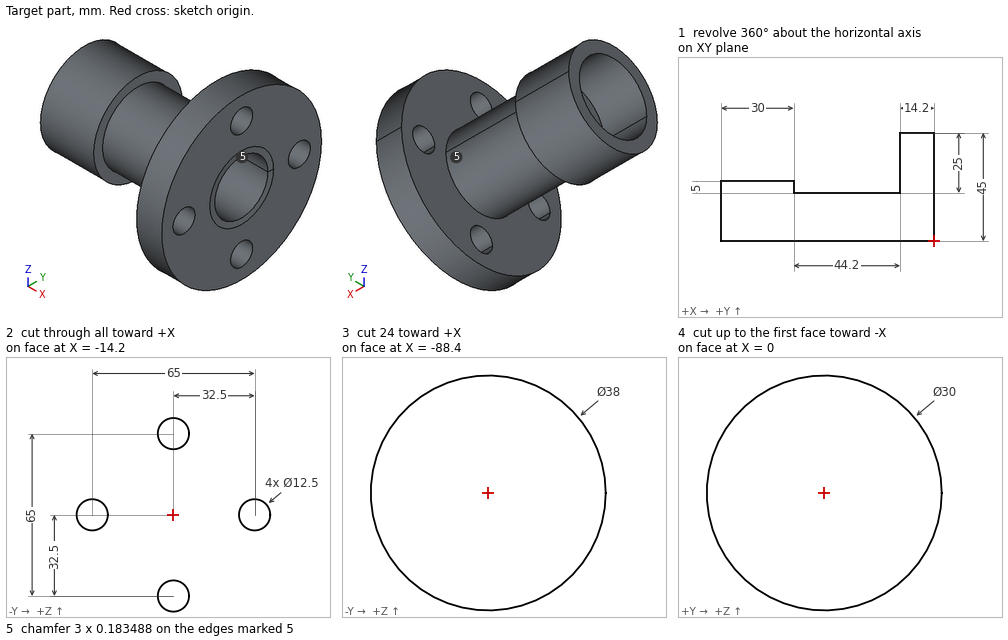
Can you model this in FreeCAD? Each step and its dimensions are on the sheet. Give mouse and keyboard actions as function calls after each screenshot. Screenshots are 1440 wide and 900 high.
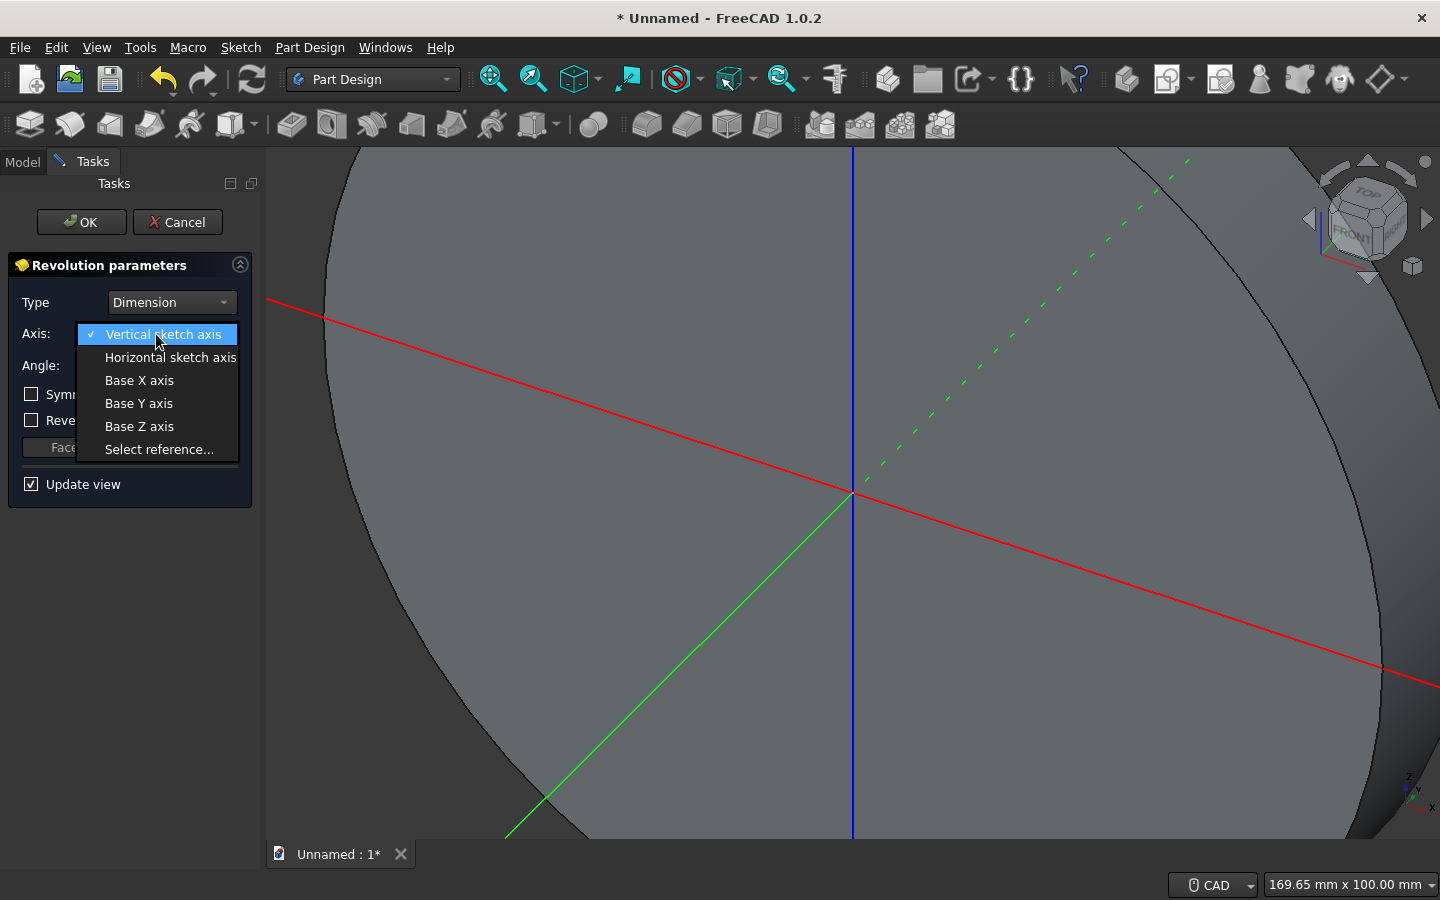
click(156, 358)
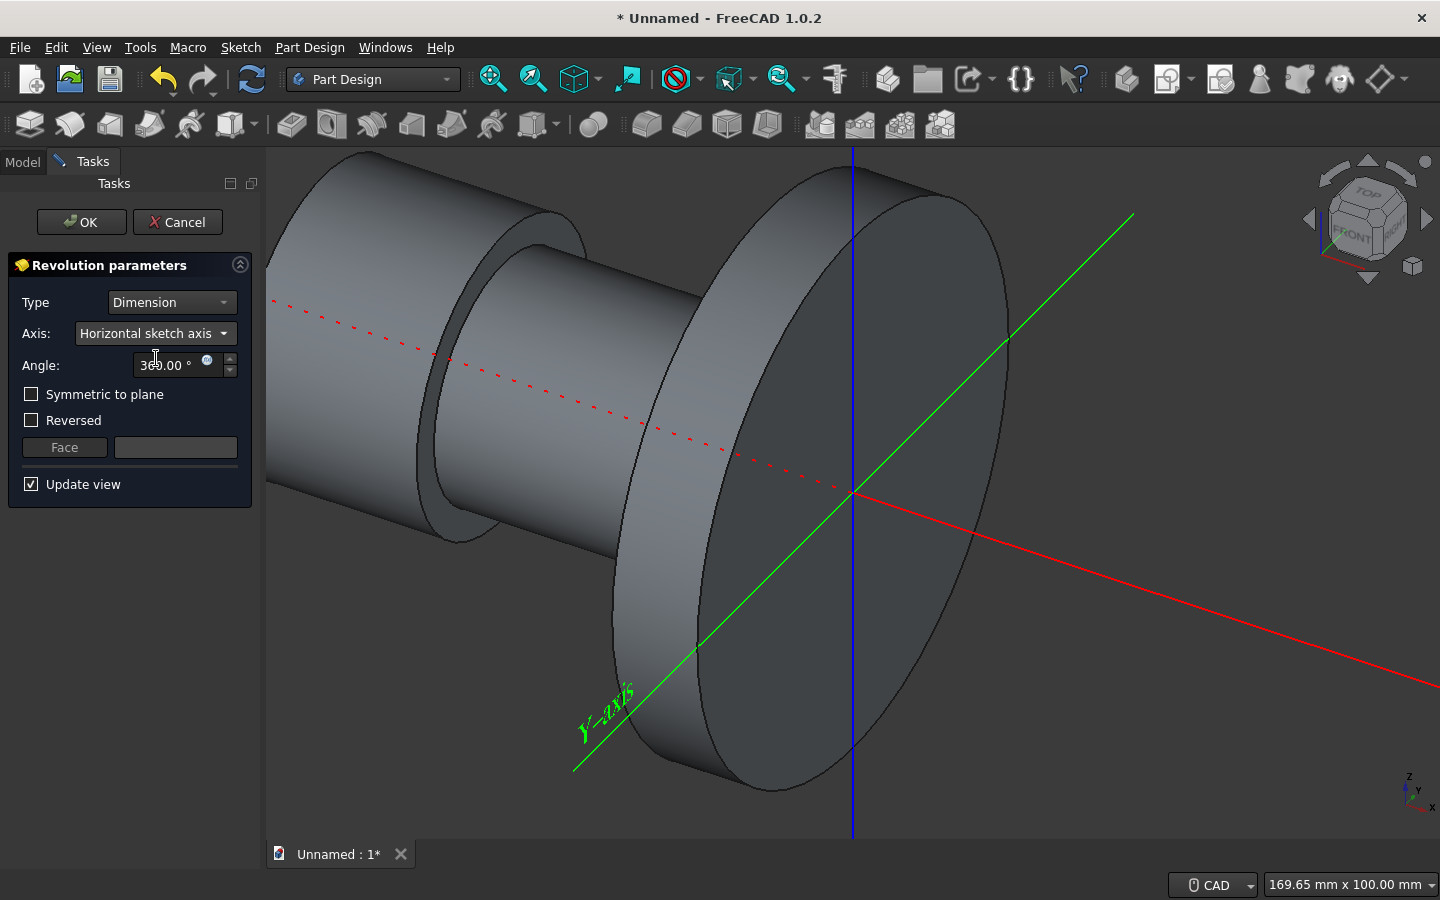
click(82, 222)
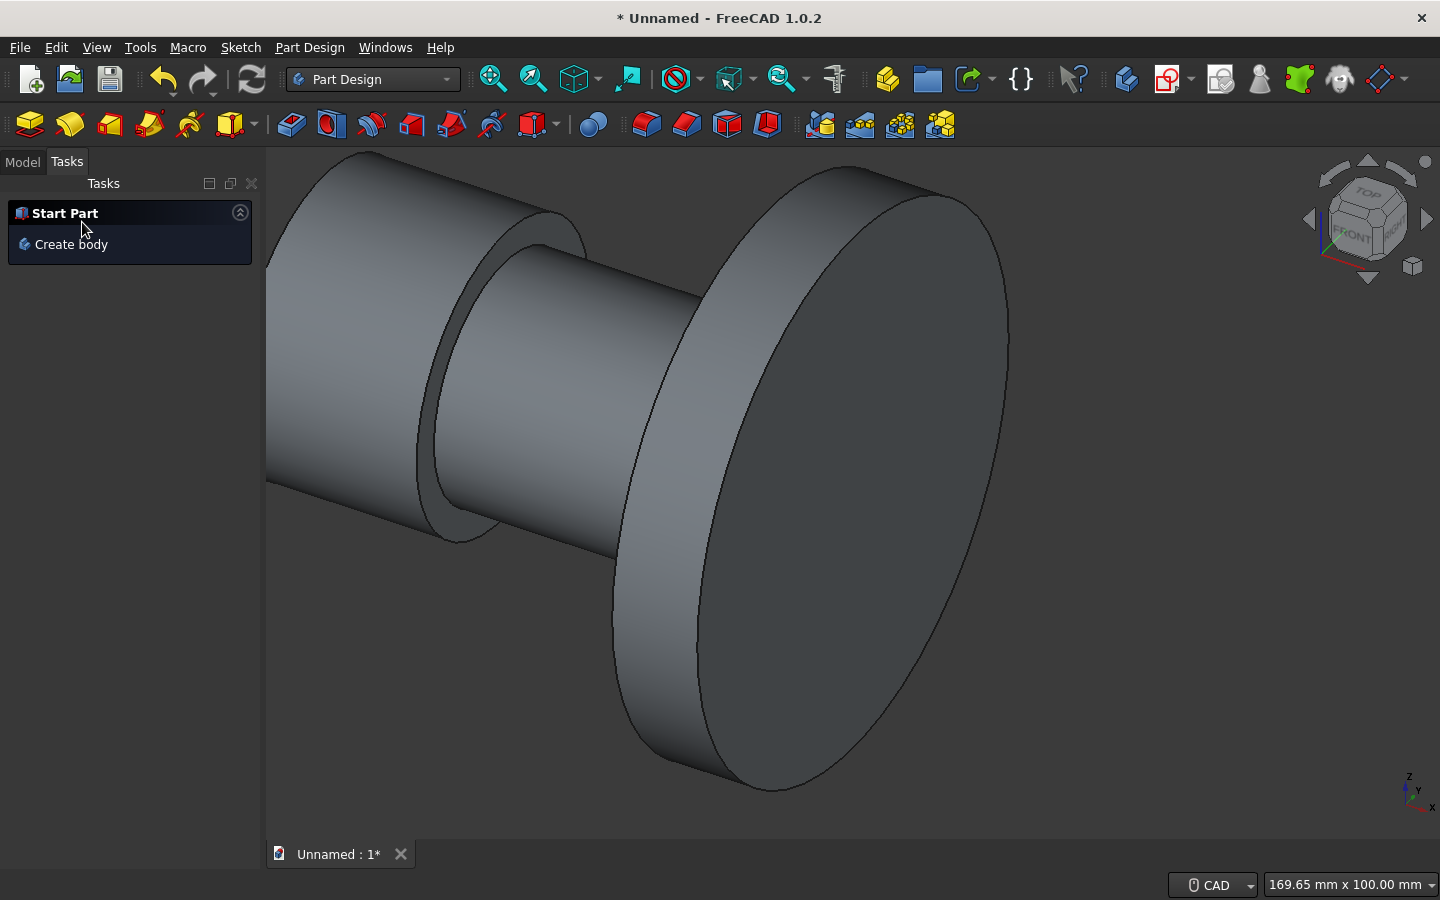
key(v)
key(f)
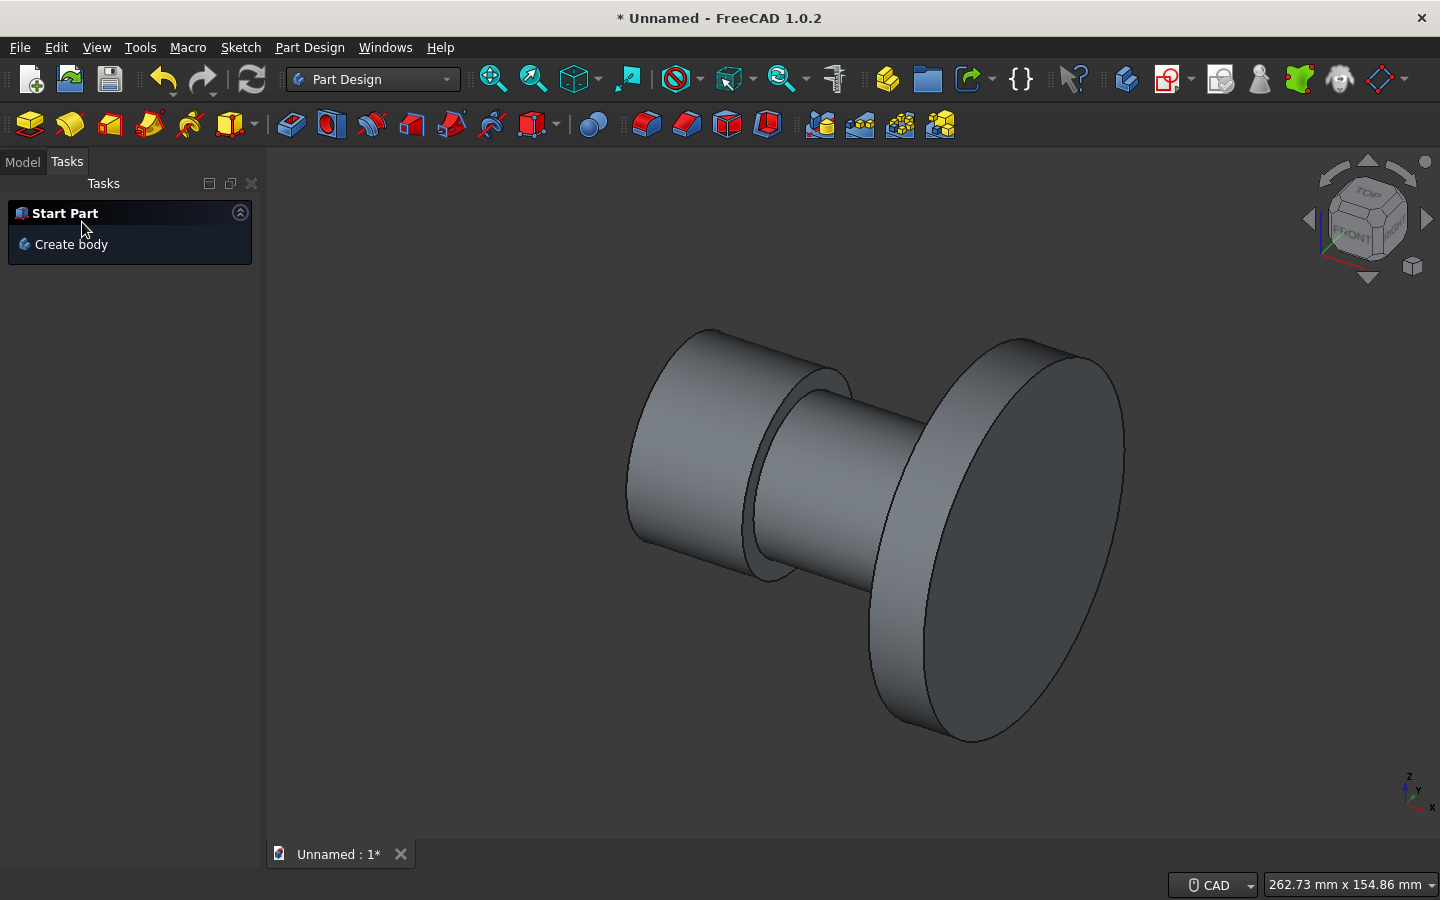
key(6)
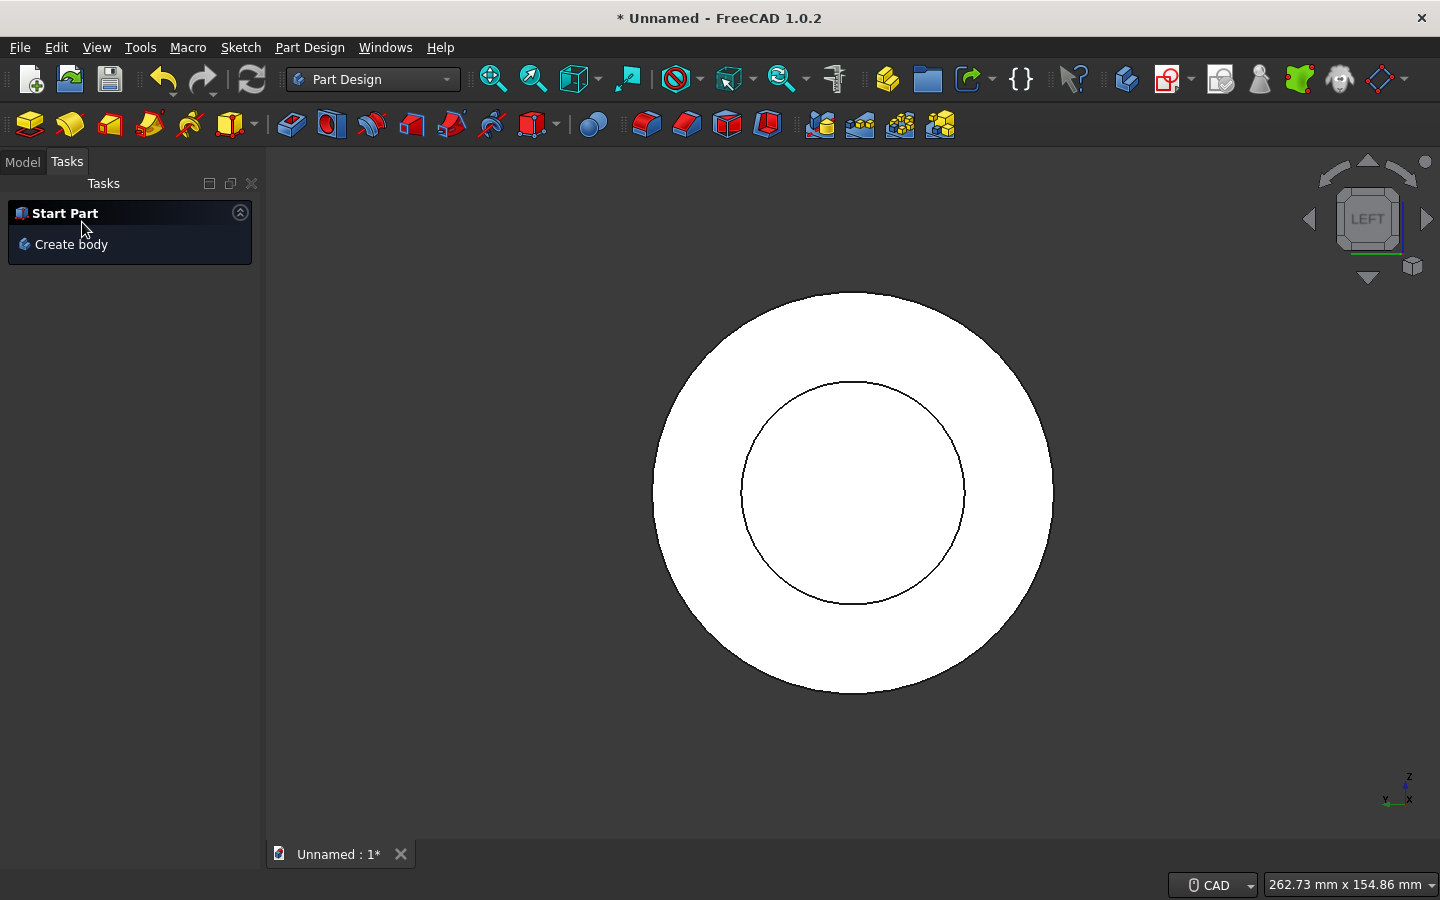
click(796, 607)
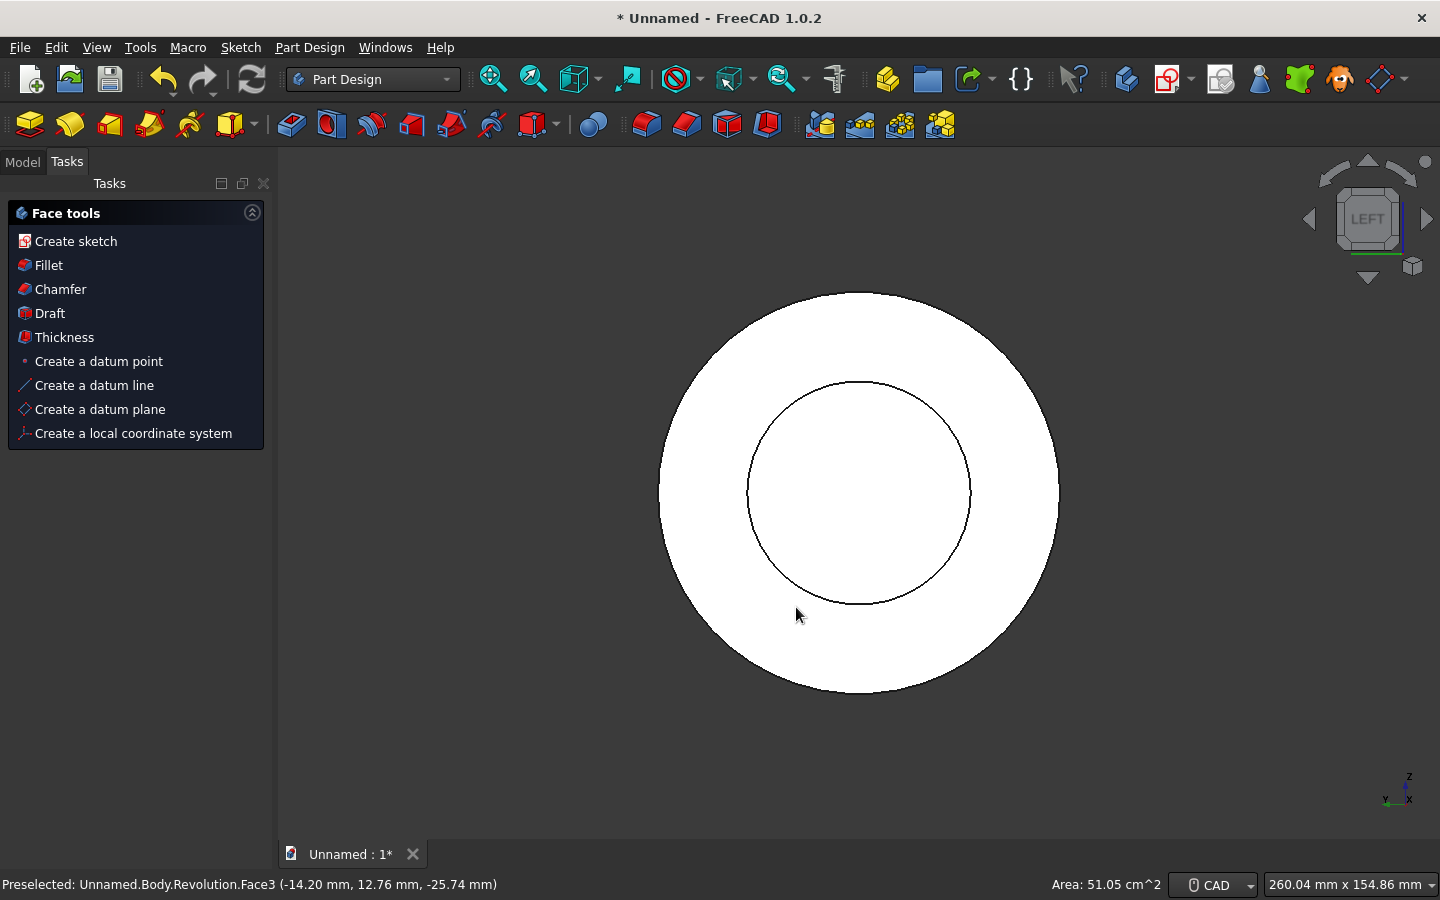
click(1168, 80)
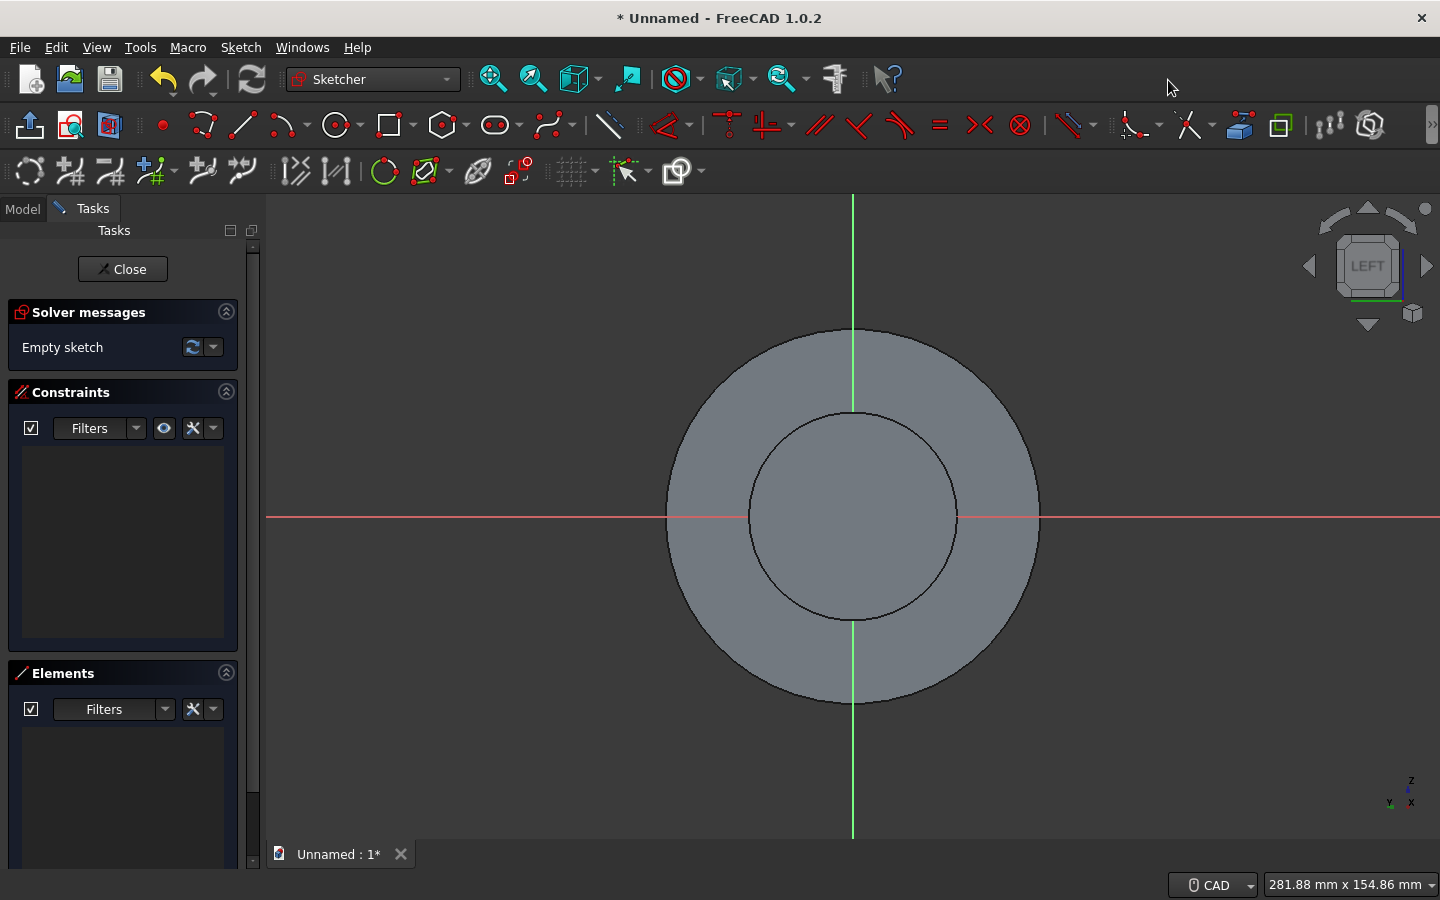
key(g)
key(c)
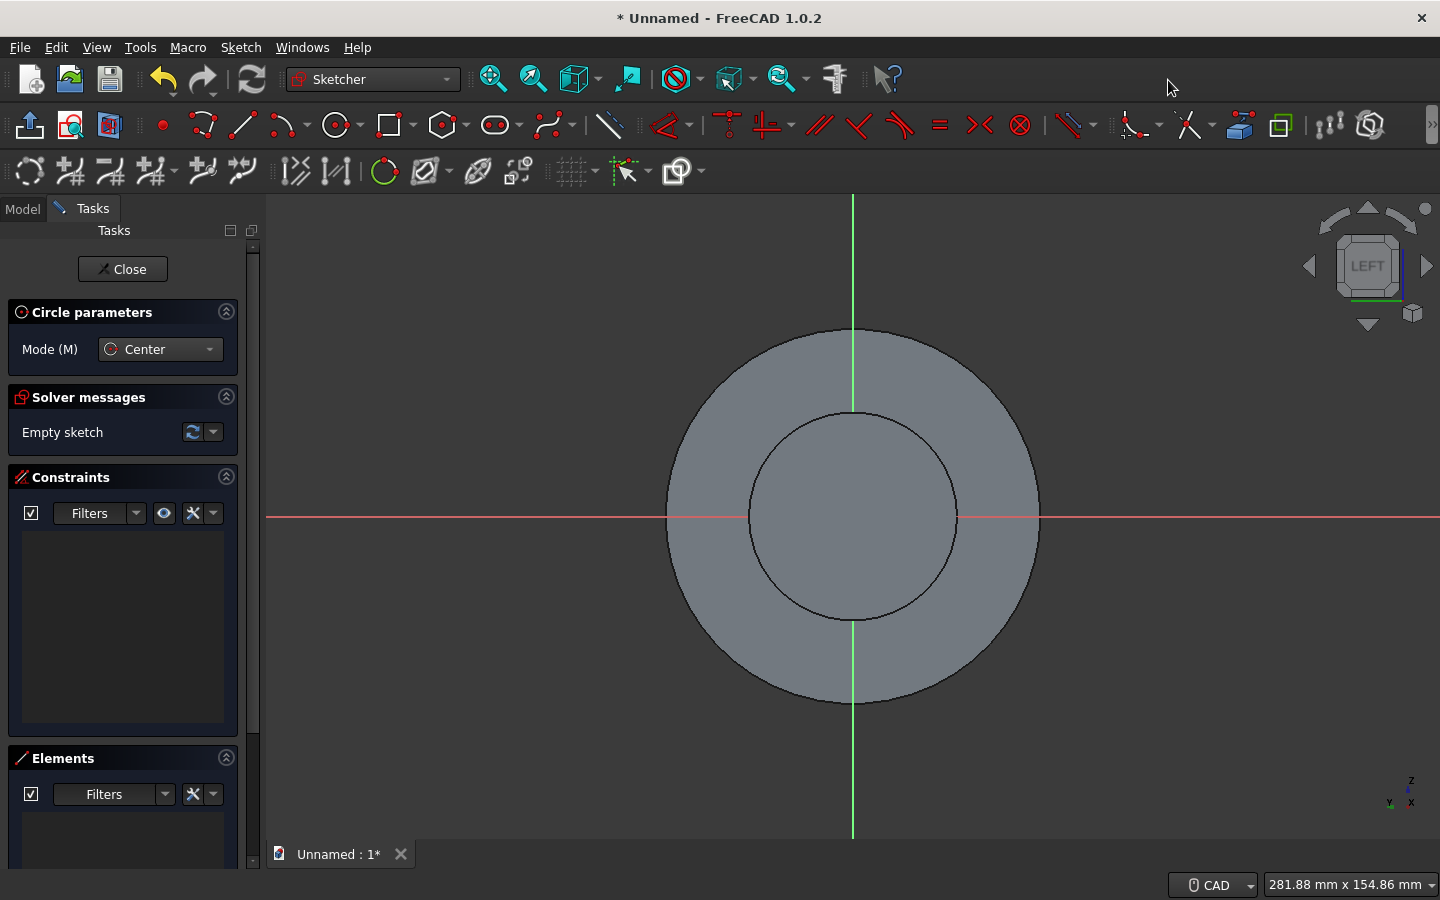
click(988, 516)
click(1007, 498)